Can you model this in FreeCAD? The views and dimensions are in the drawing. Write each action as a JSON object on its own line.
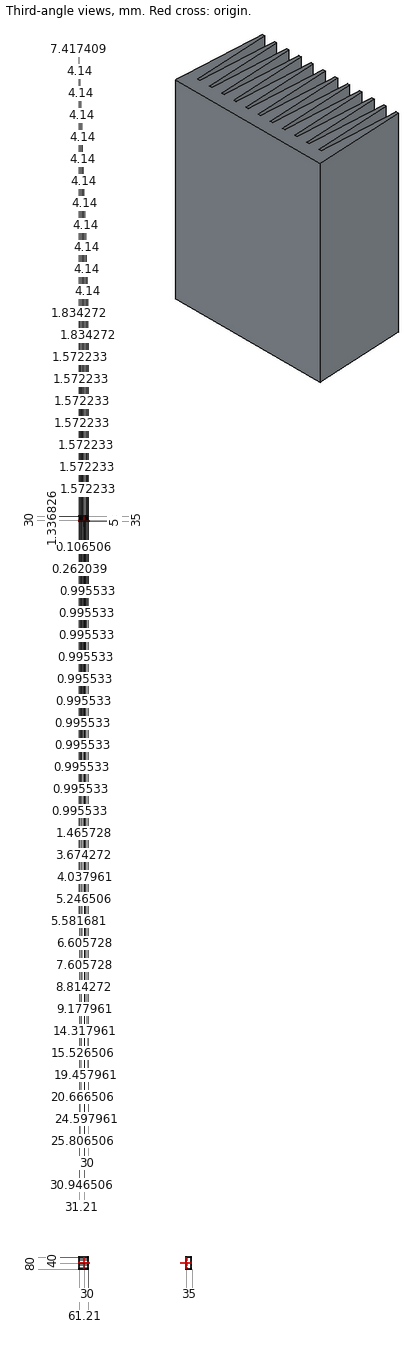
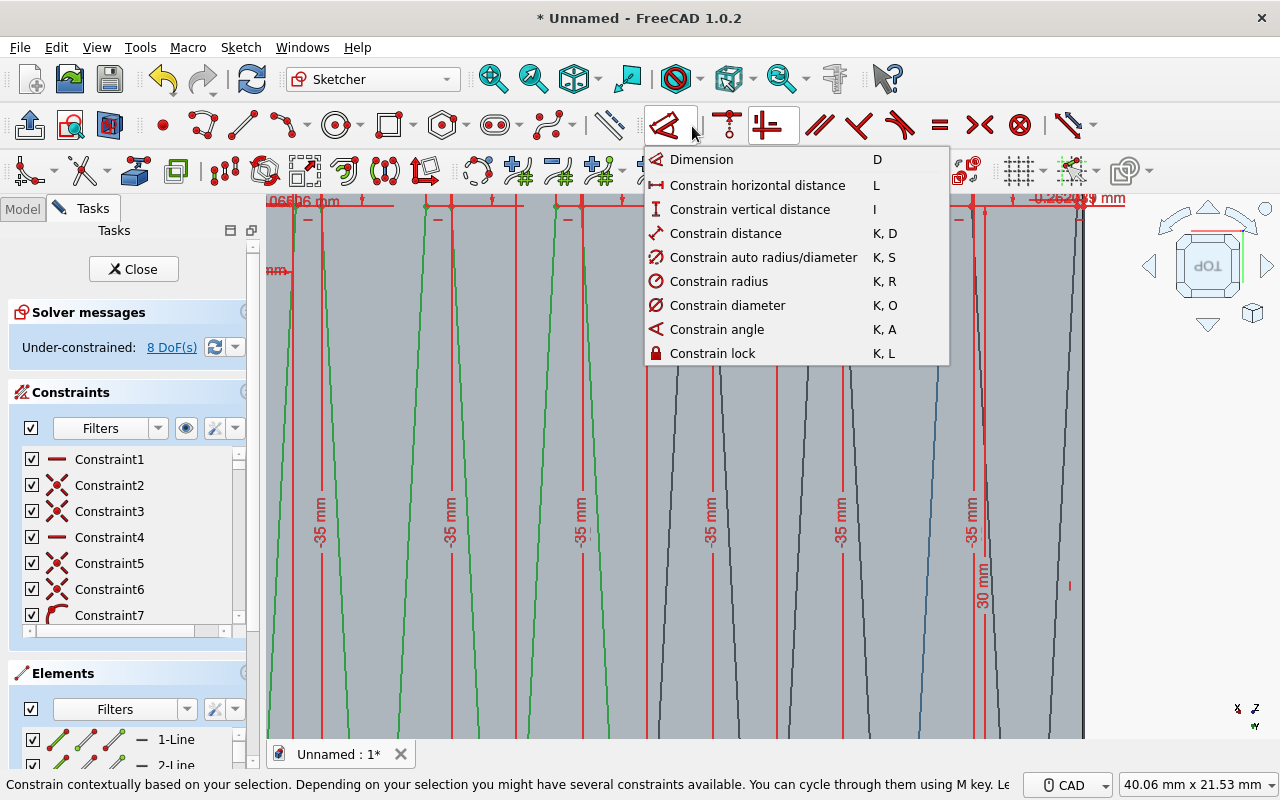
{"action": "left_click", "coordinate": [797, 185]}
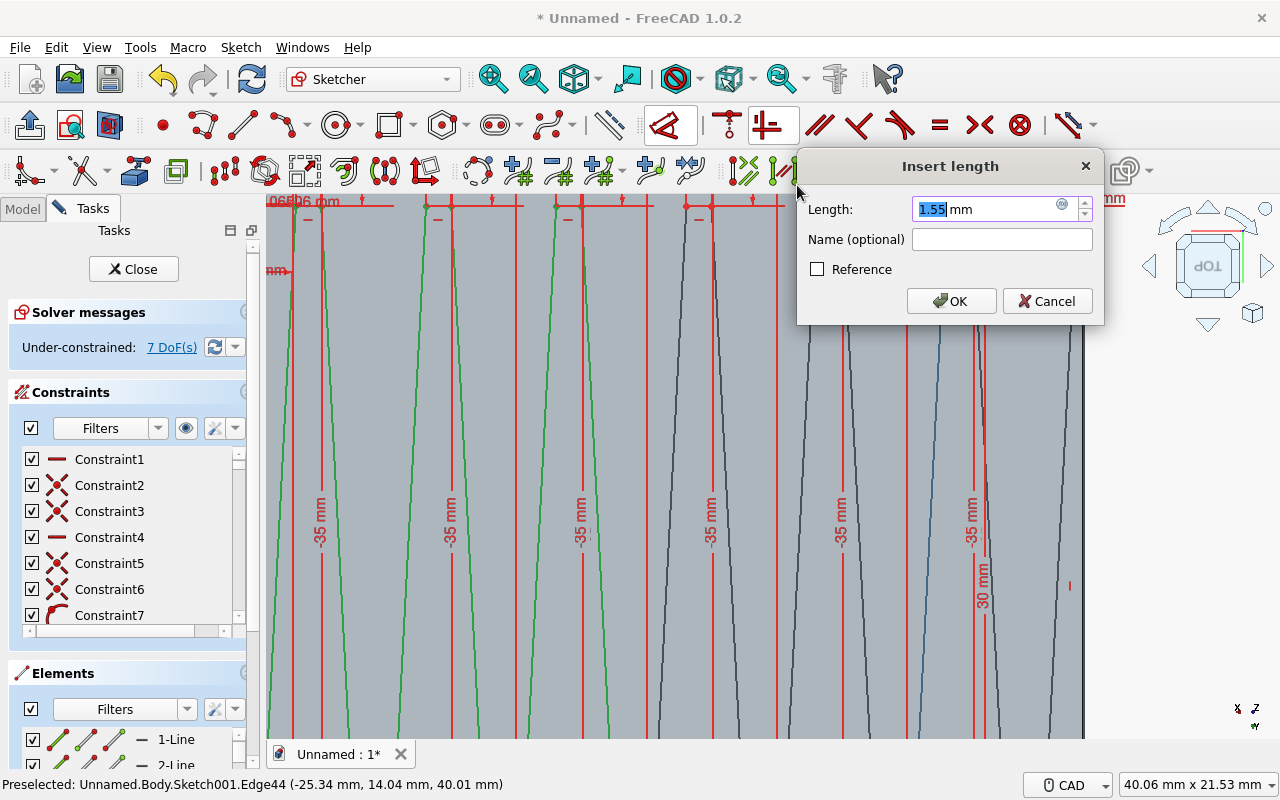
{"action": "type", "text": "1.572233"}
{"action": "key", "text": "Return"}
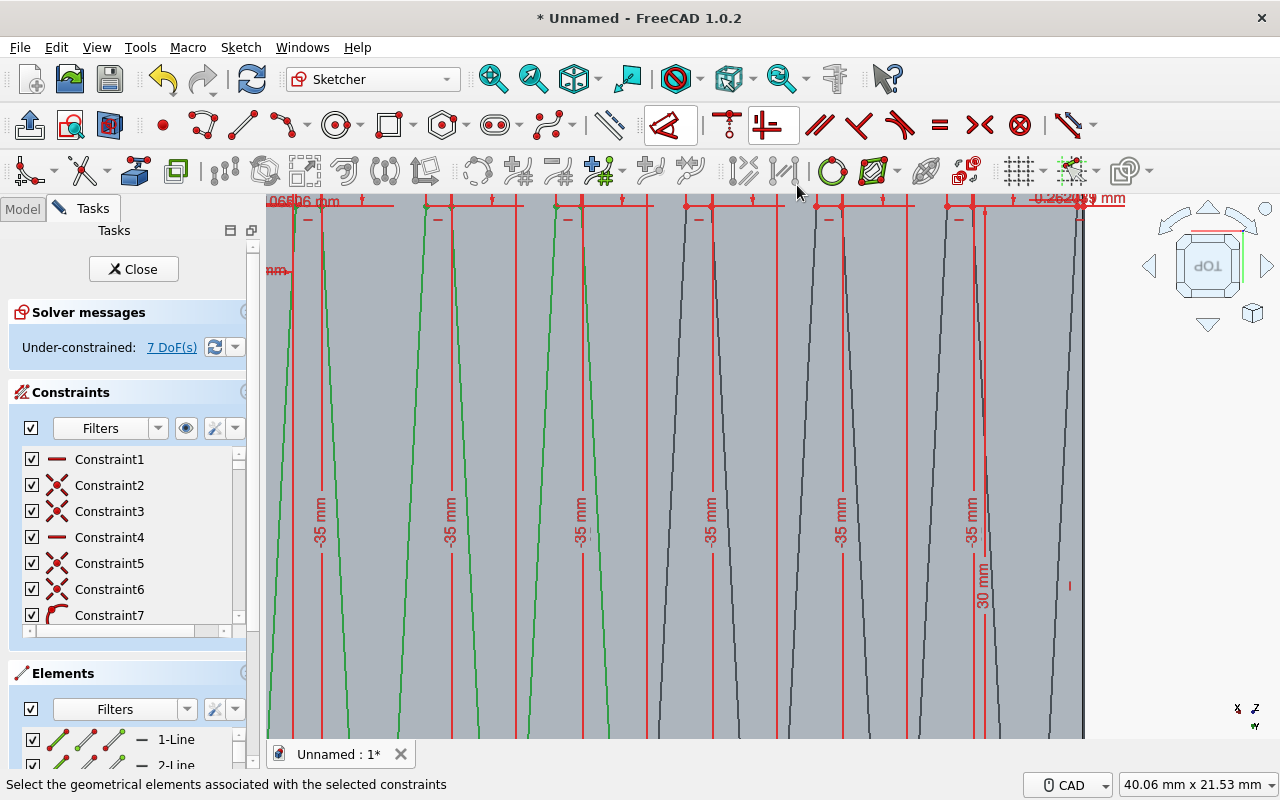
{"action": "scroll", "coordinate": [935, 434], "scroll_direction": "down", "scroll_amount": 5}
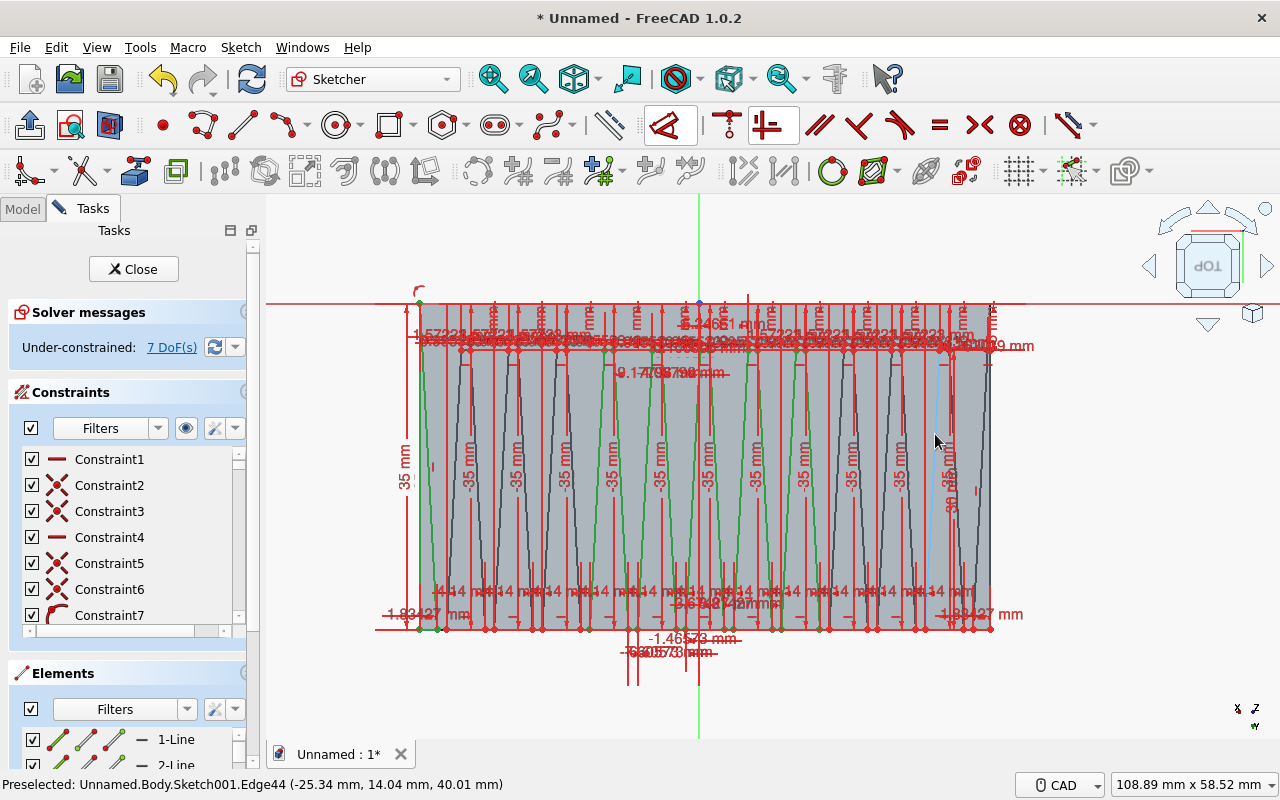
{"action": "scroll", "coordinate": [471, 350], "scroll_direction": "up", "scroll_amount": 2}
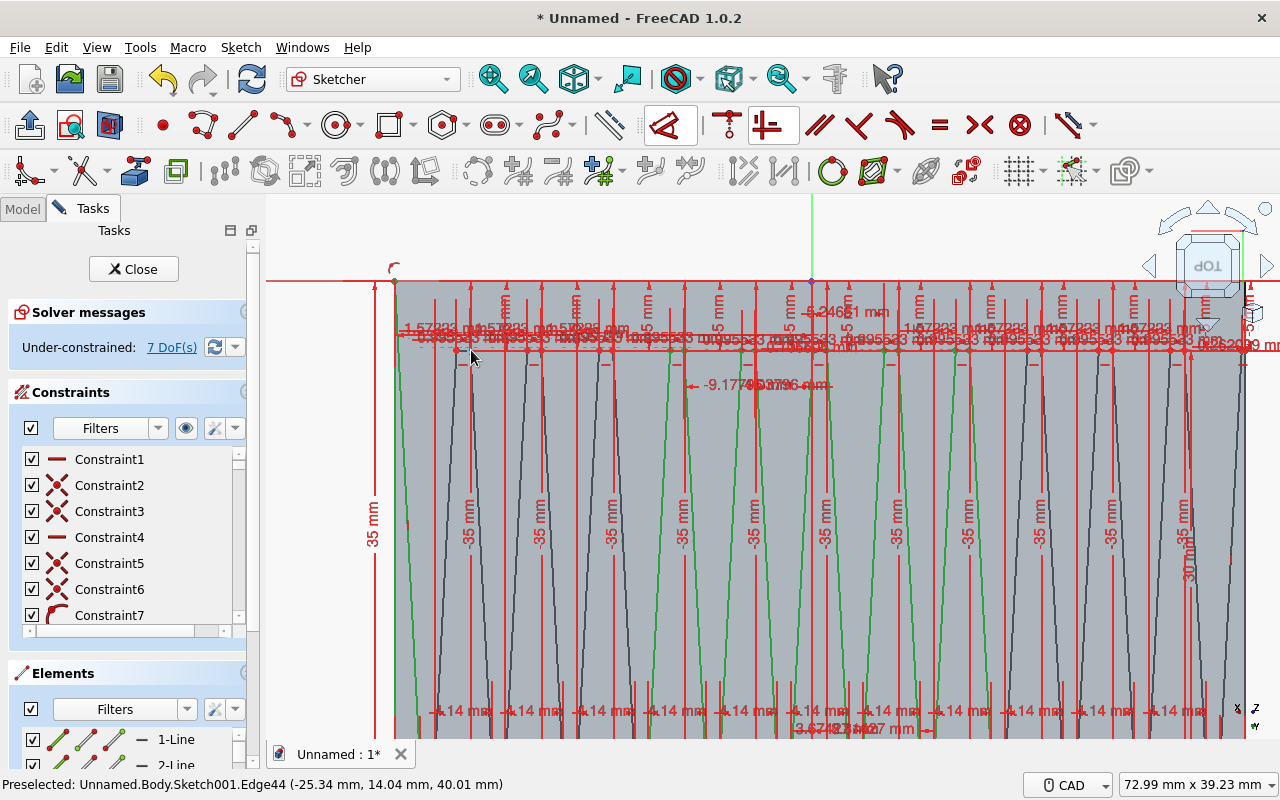
{"action": "left_click", "coordinate": [470, 351]}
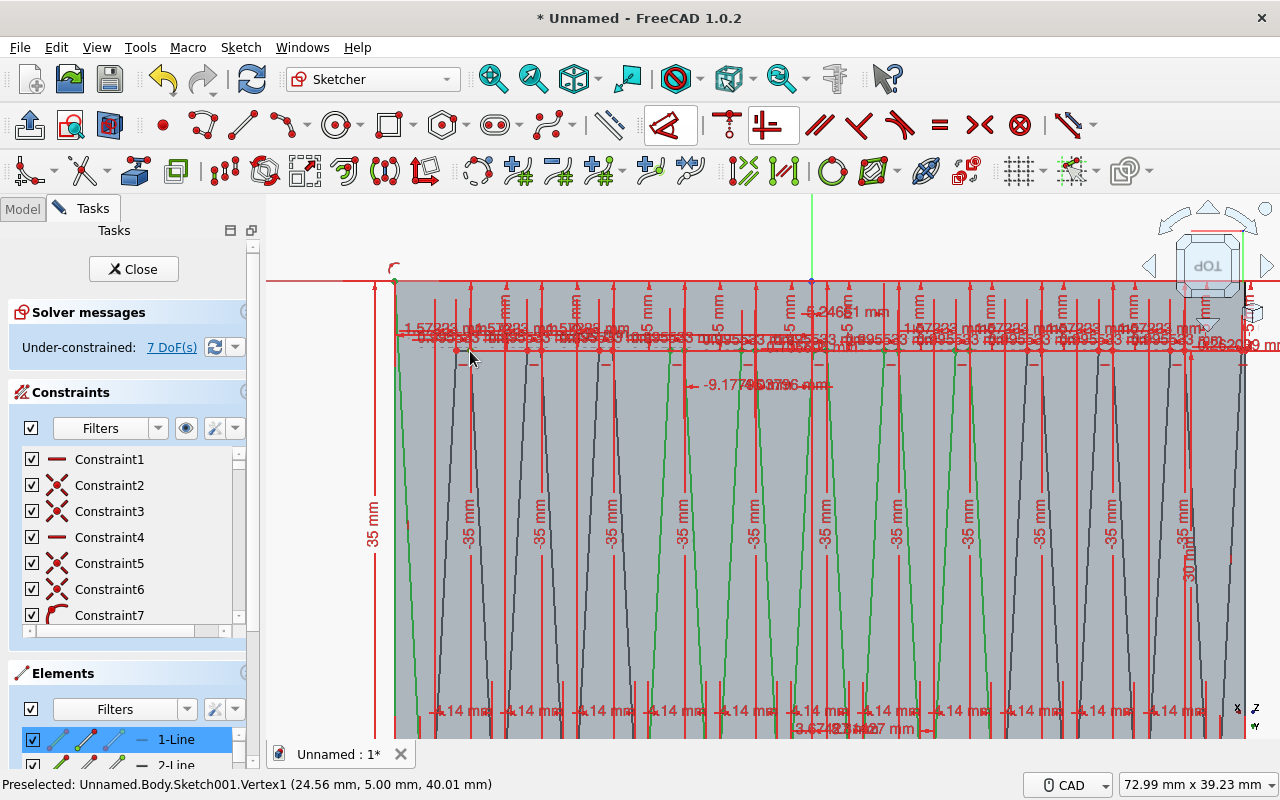
{"action": "left_click", "coordinate": [692, 126]}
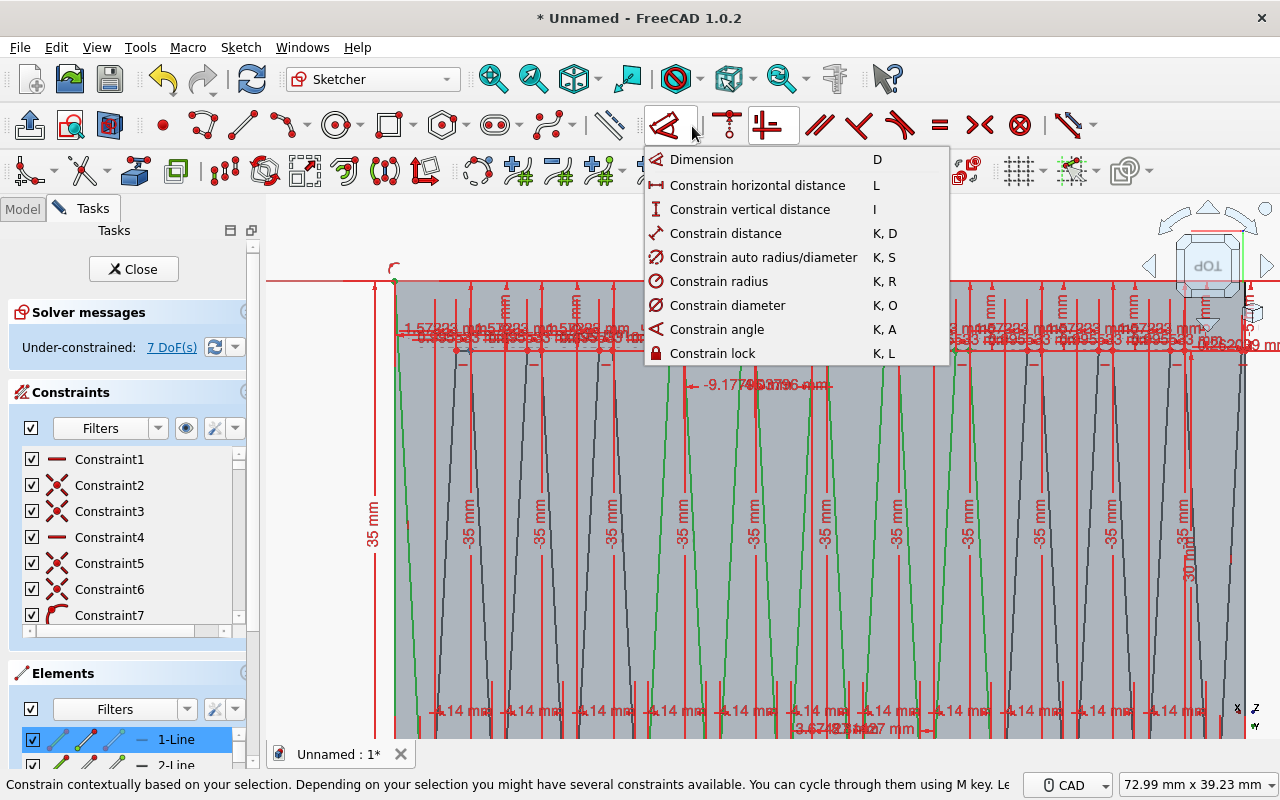
{"action": "left_click", "coordinate": [797, 185]}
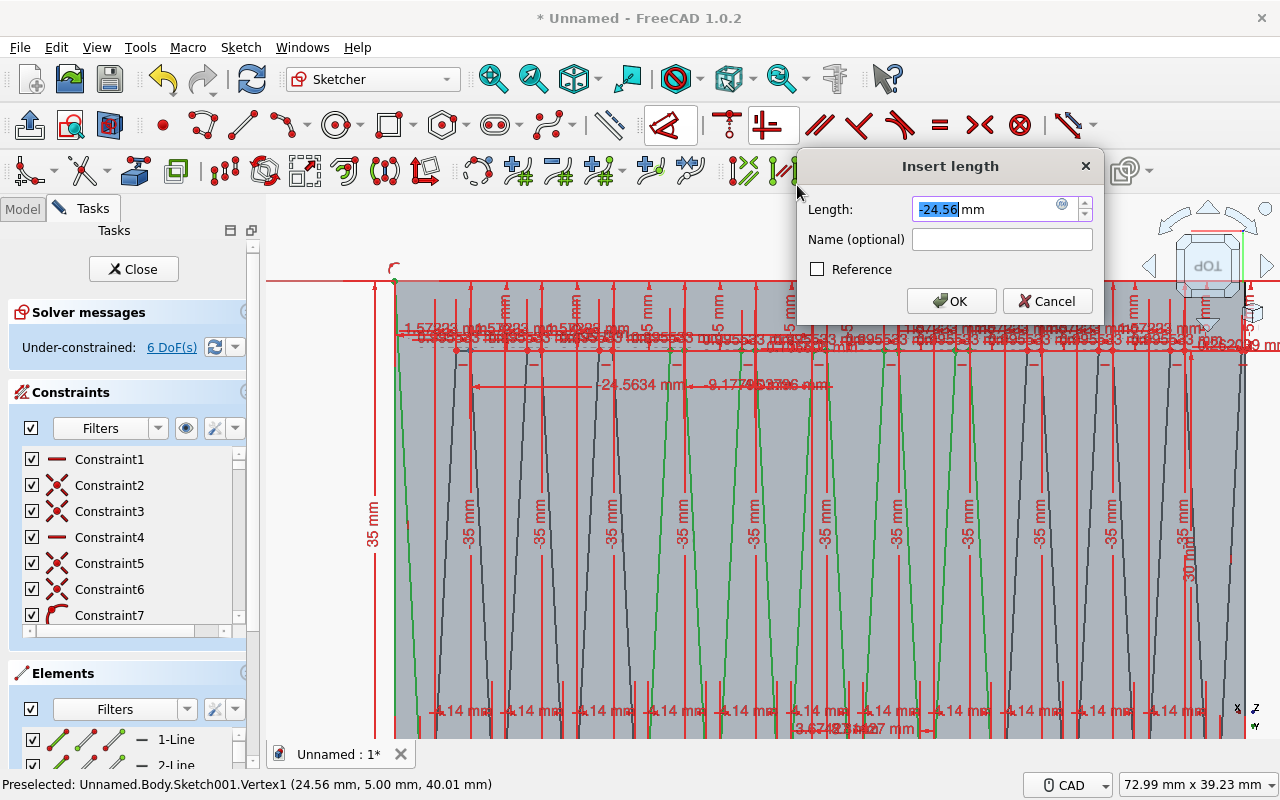
{"action": "type", "text": "-24.597961"}
{"action": "key", "text": "Return"}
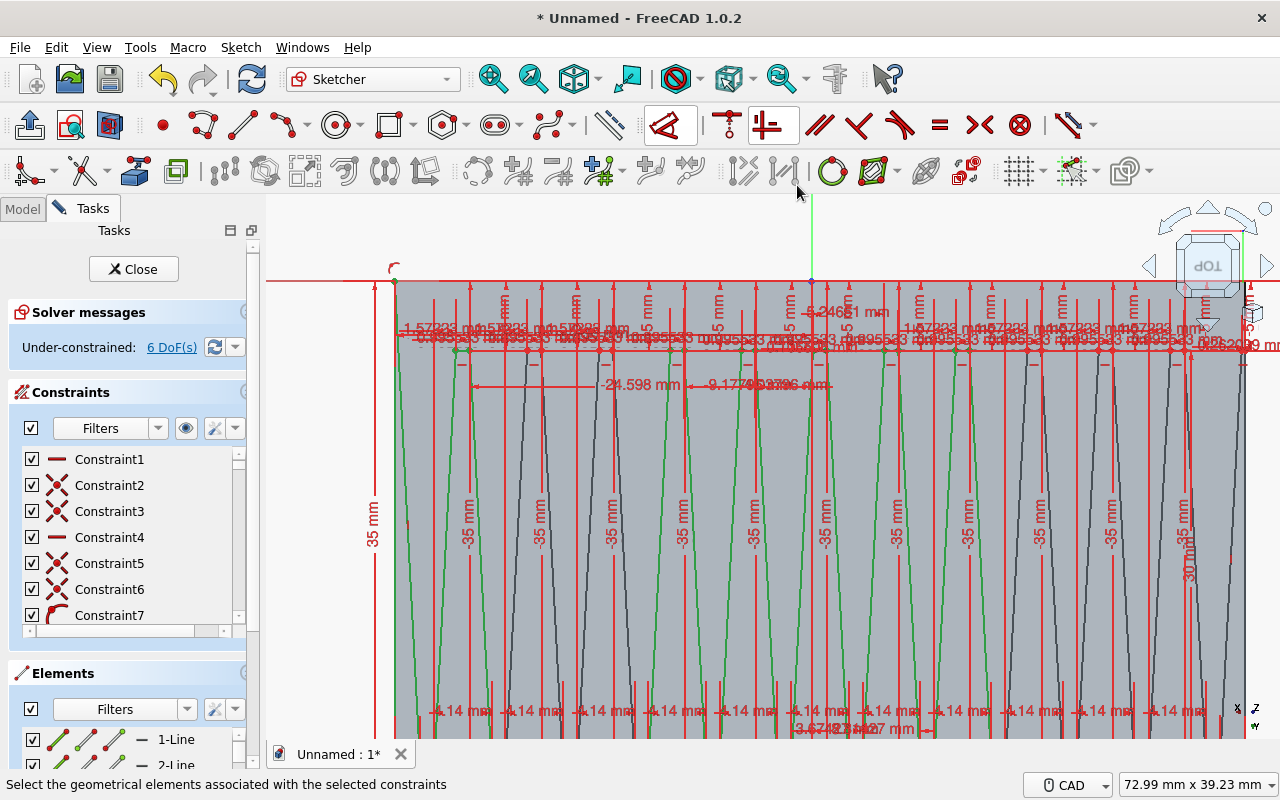
{"action": "left_click", "coordinate": [541, 351]}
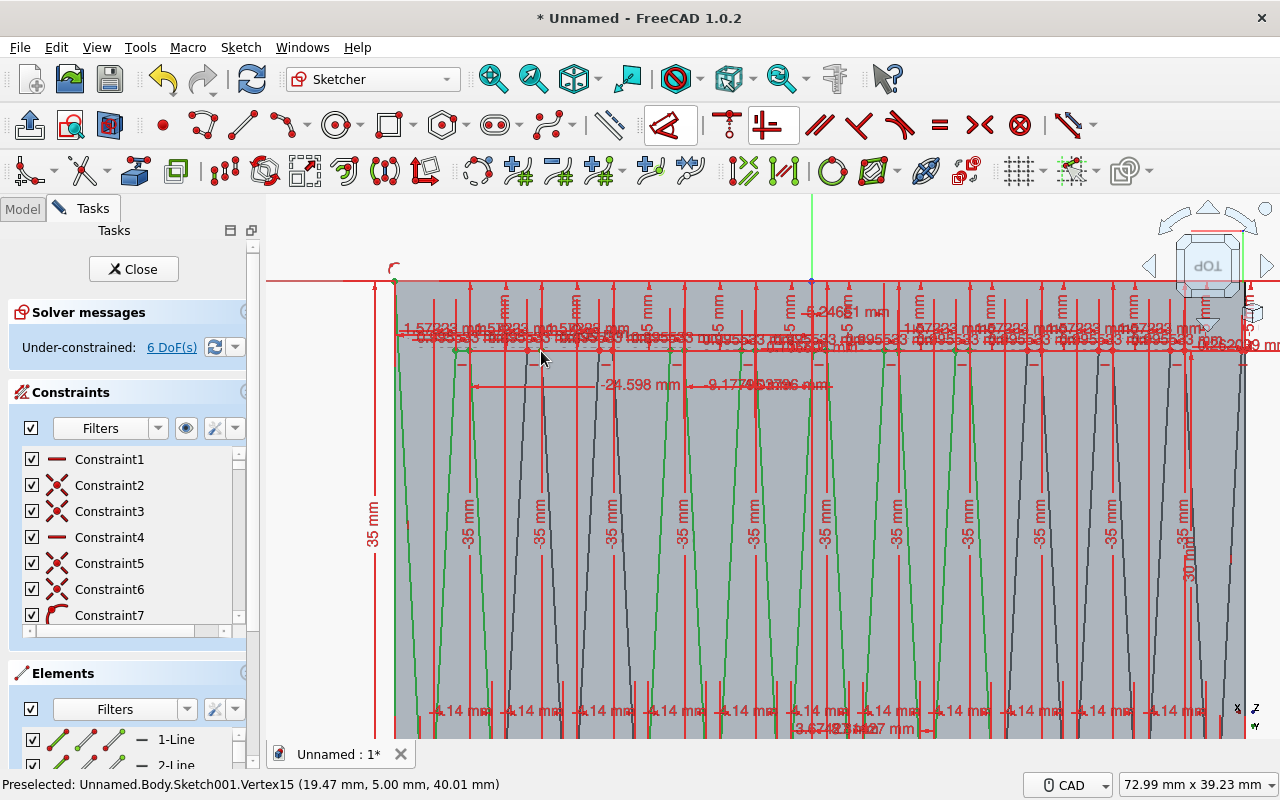
{"action": "left_click", "coordinate": [692, 126]}